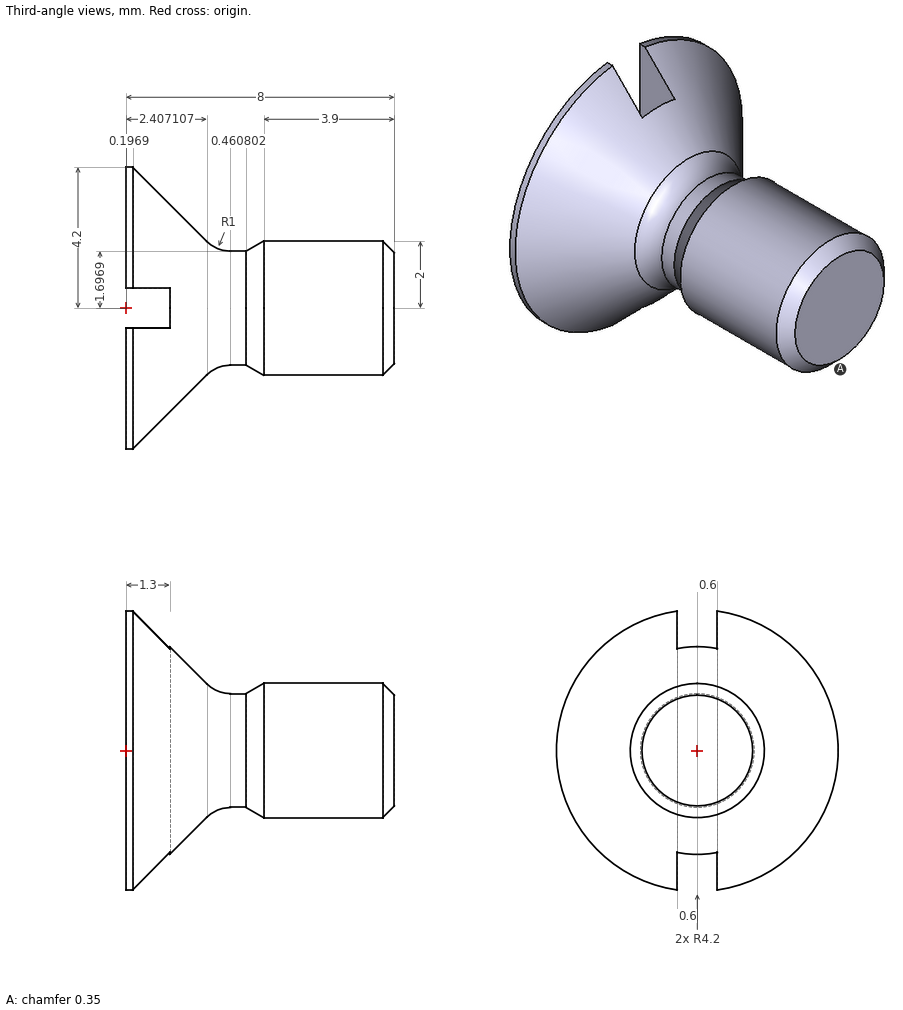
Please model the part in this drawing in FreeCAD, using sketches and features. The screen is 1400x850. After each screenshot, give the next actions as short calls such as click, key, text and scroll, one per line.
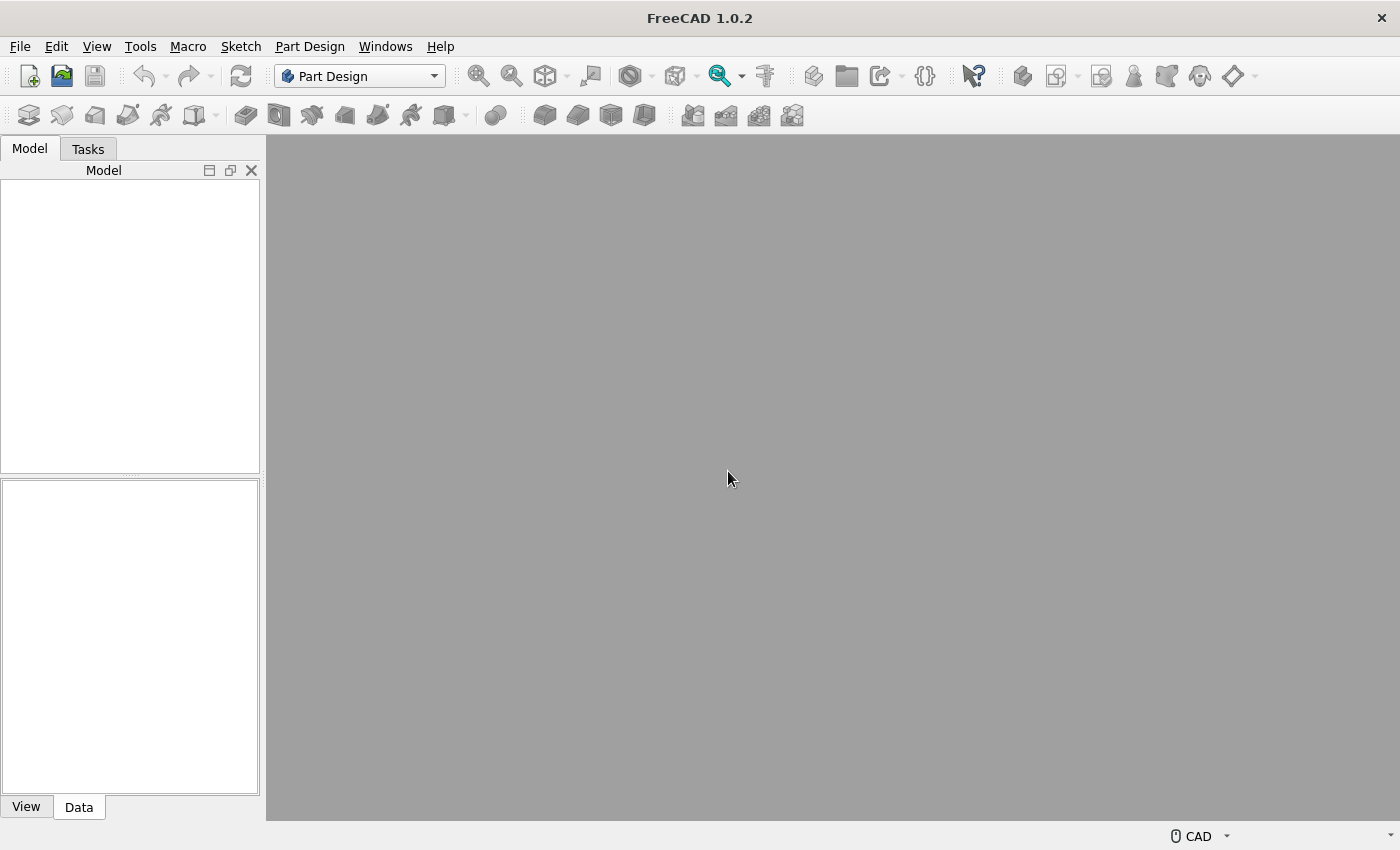
key(ctrl+n)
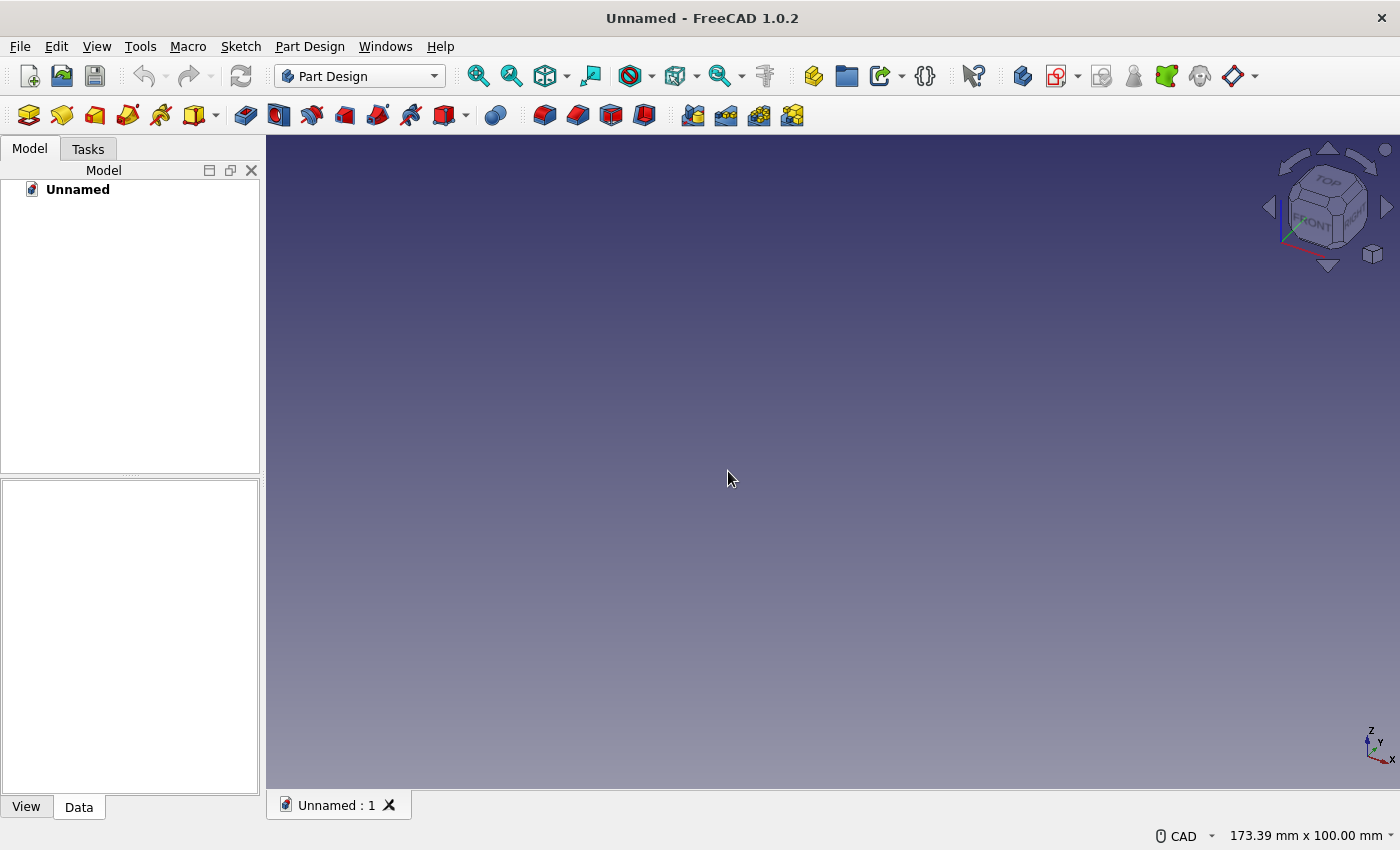
click(1056, 76)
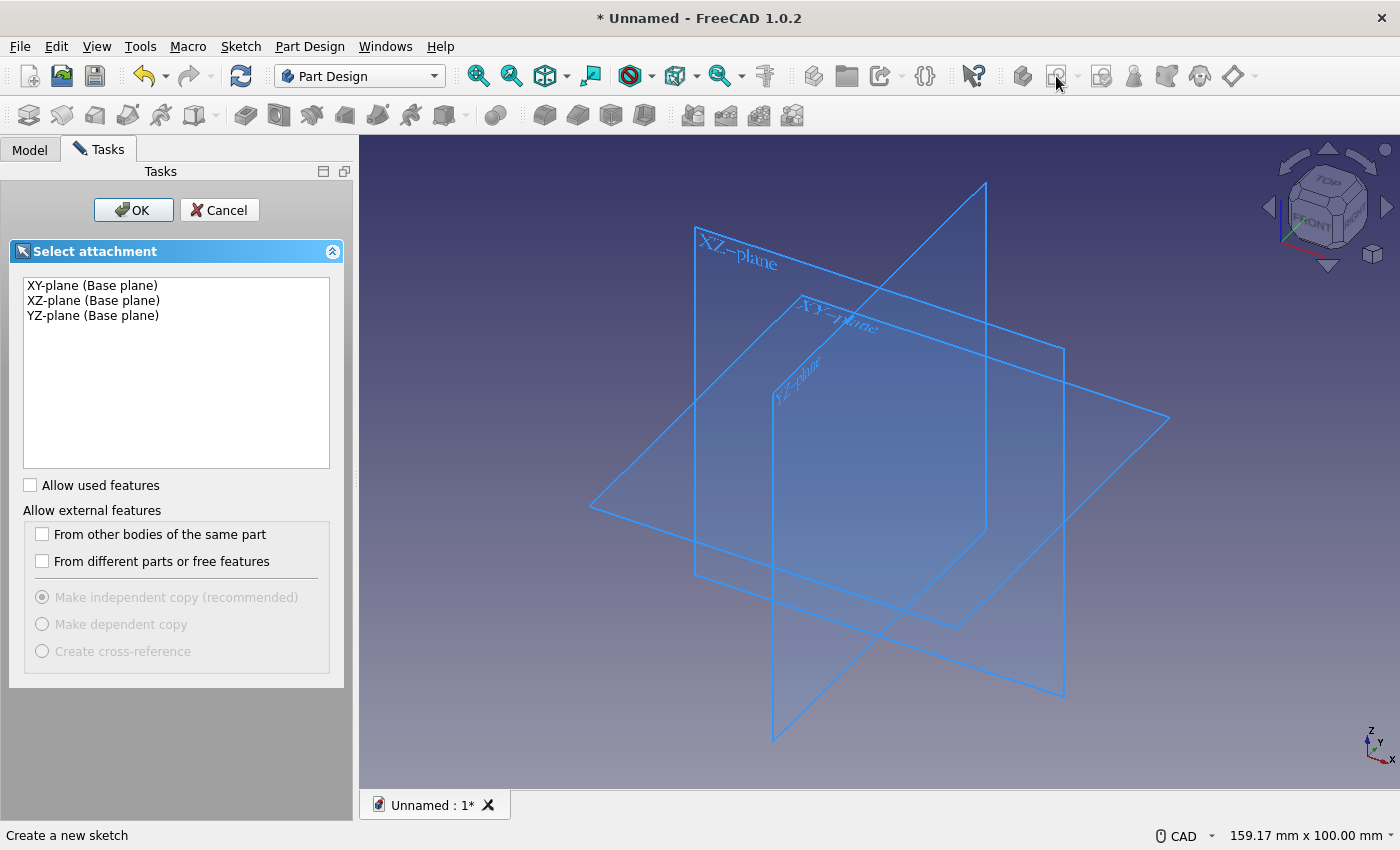
click(84, 286)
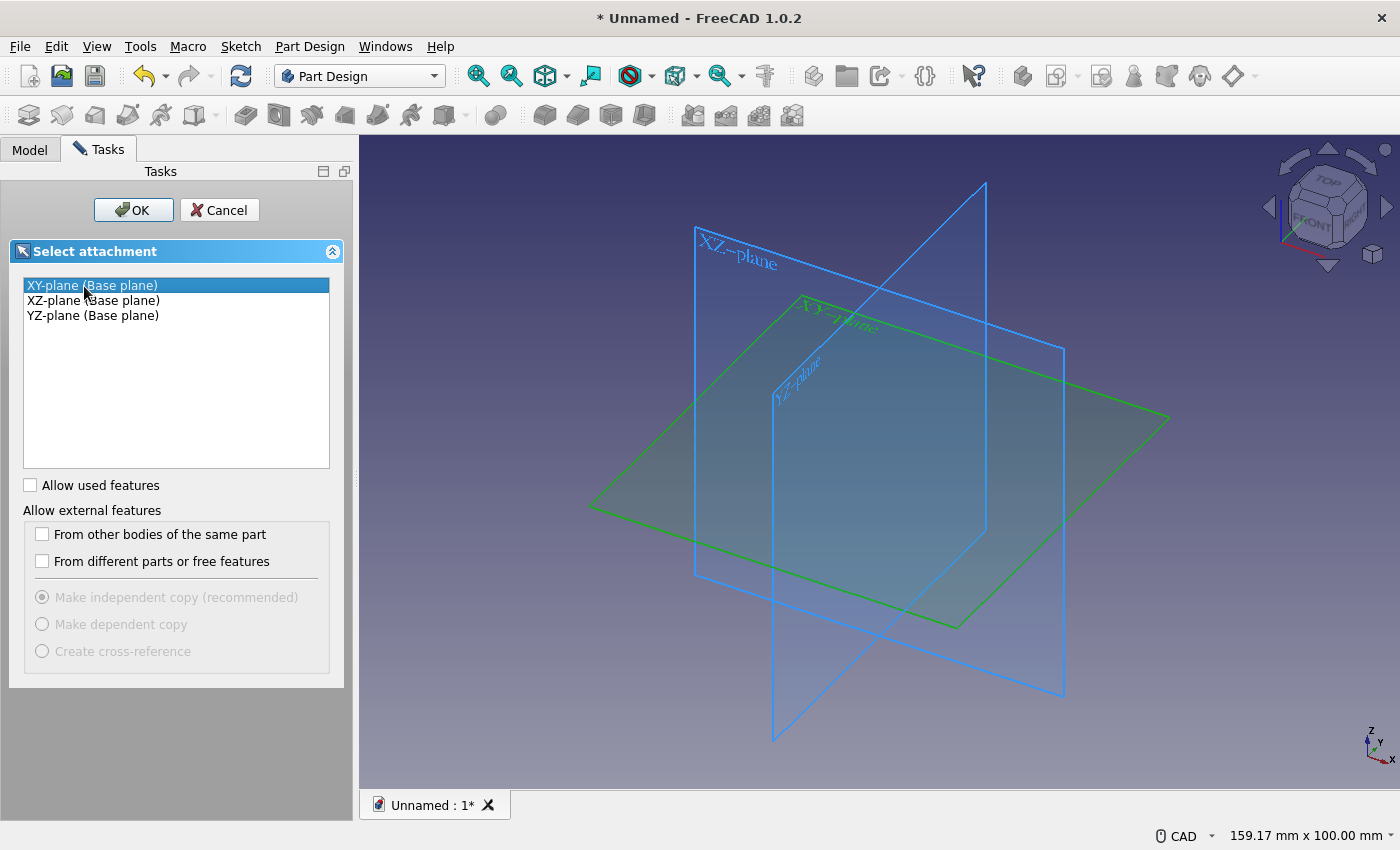
click(134, 210)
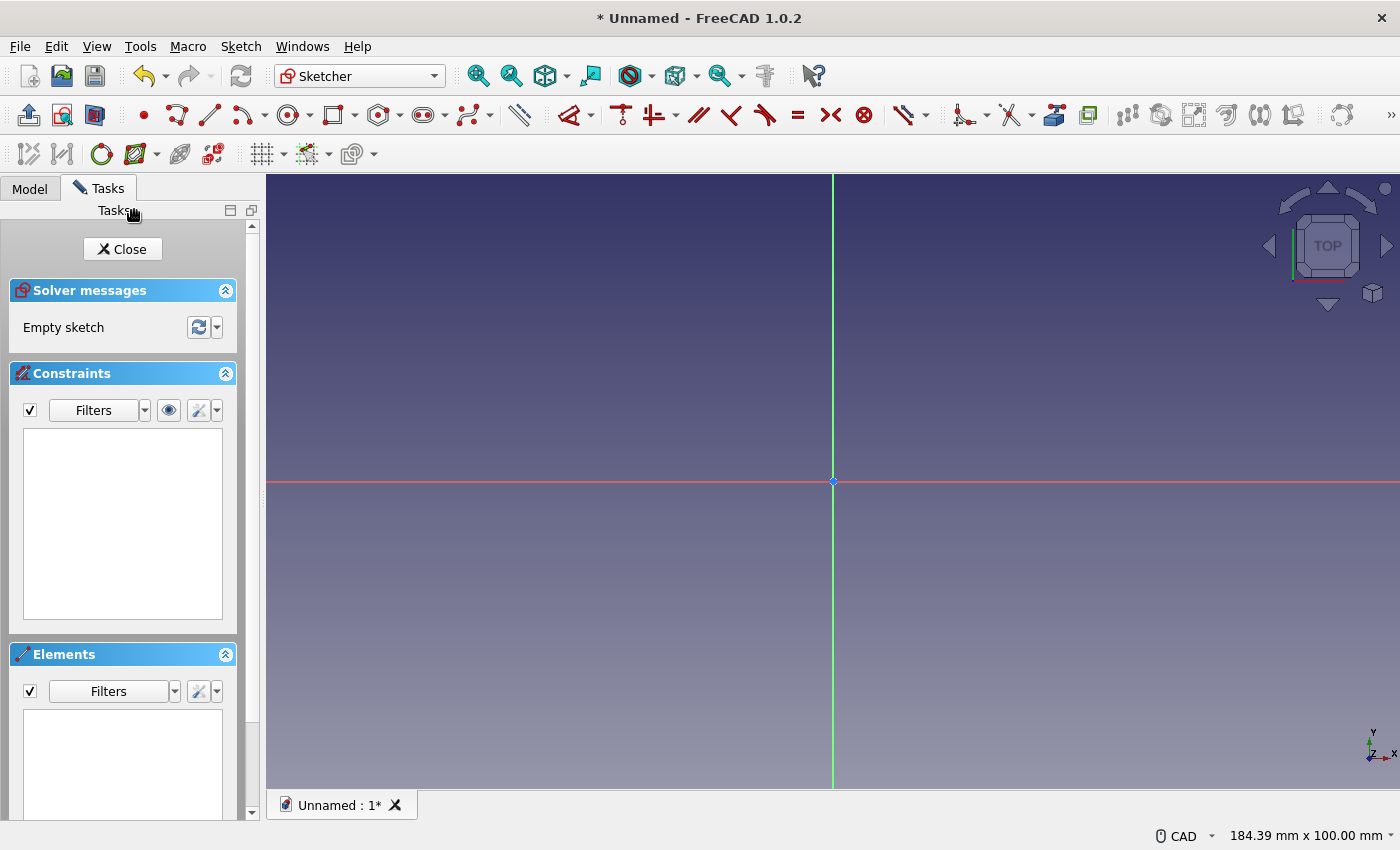
scroll(865, 468, up, 13)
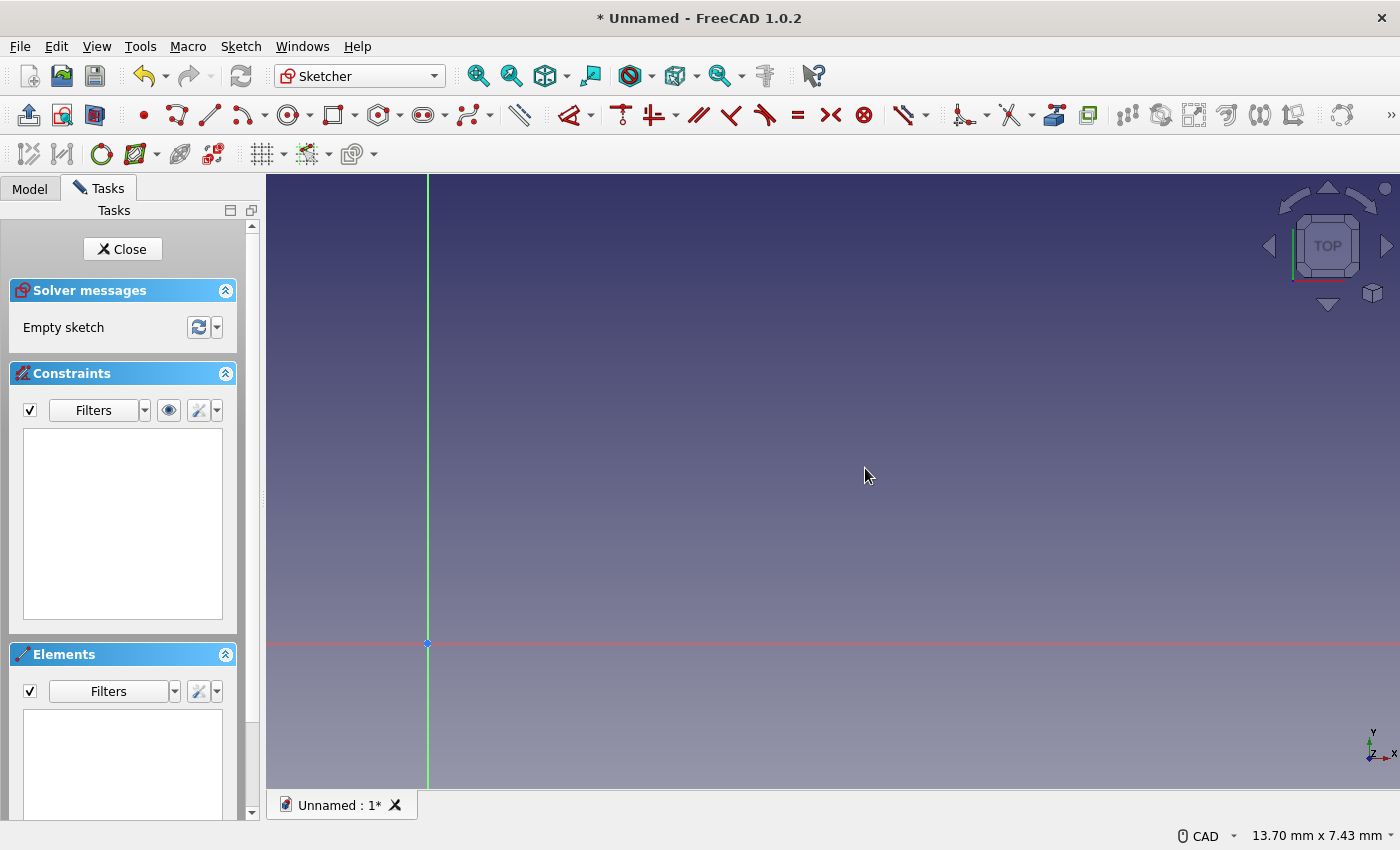
click(177, 116)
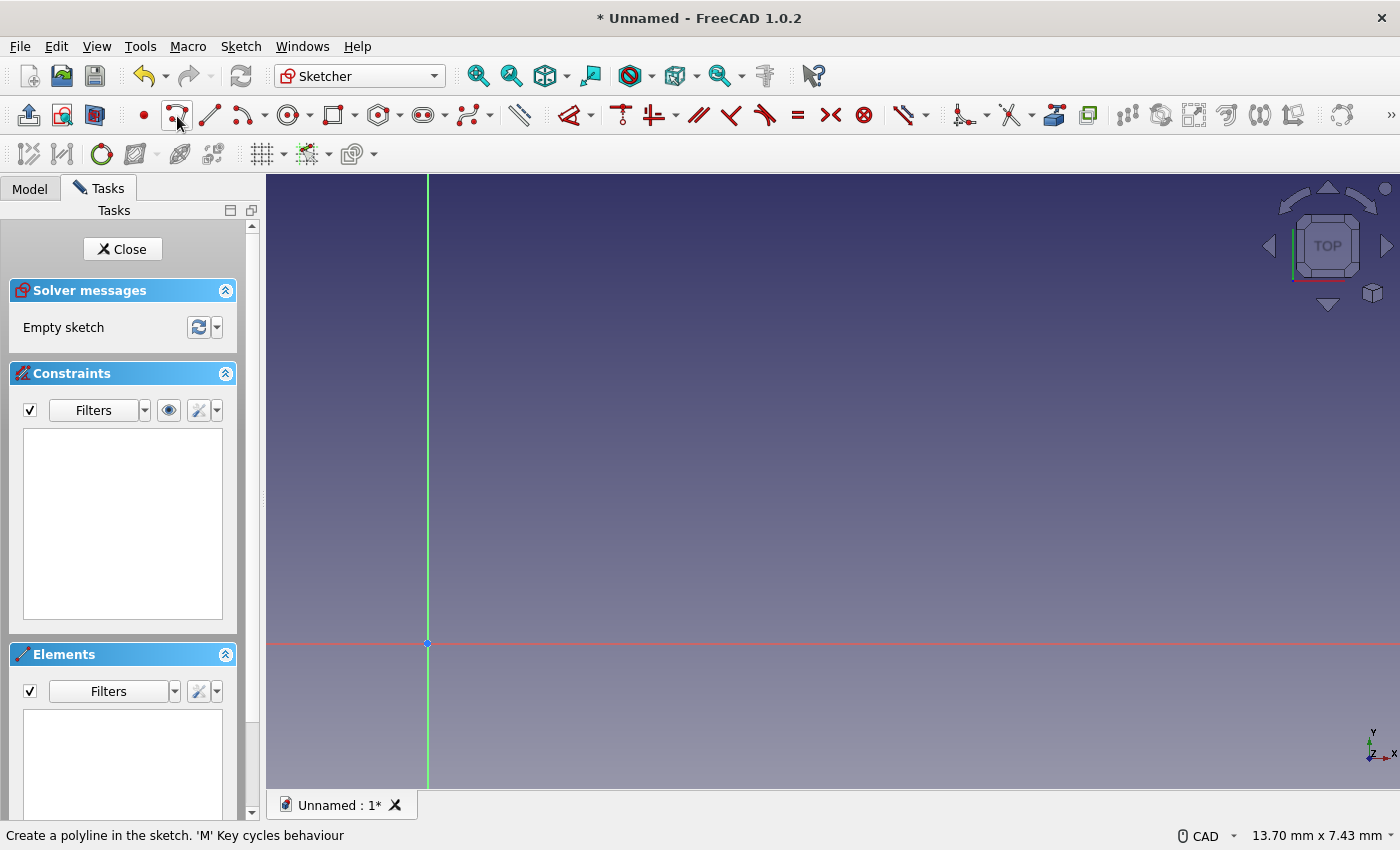
click(627, 479)
click(444, 296)
click(428, 296)
click(428, 644)
click(1090, 635)
click(1090, 478)
click(767, 478)
click(724, 503)
click(685, 503)
right_click(685, 503)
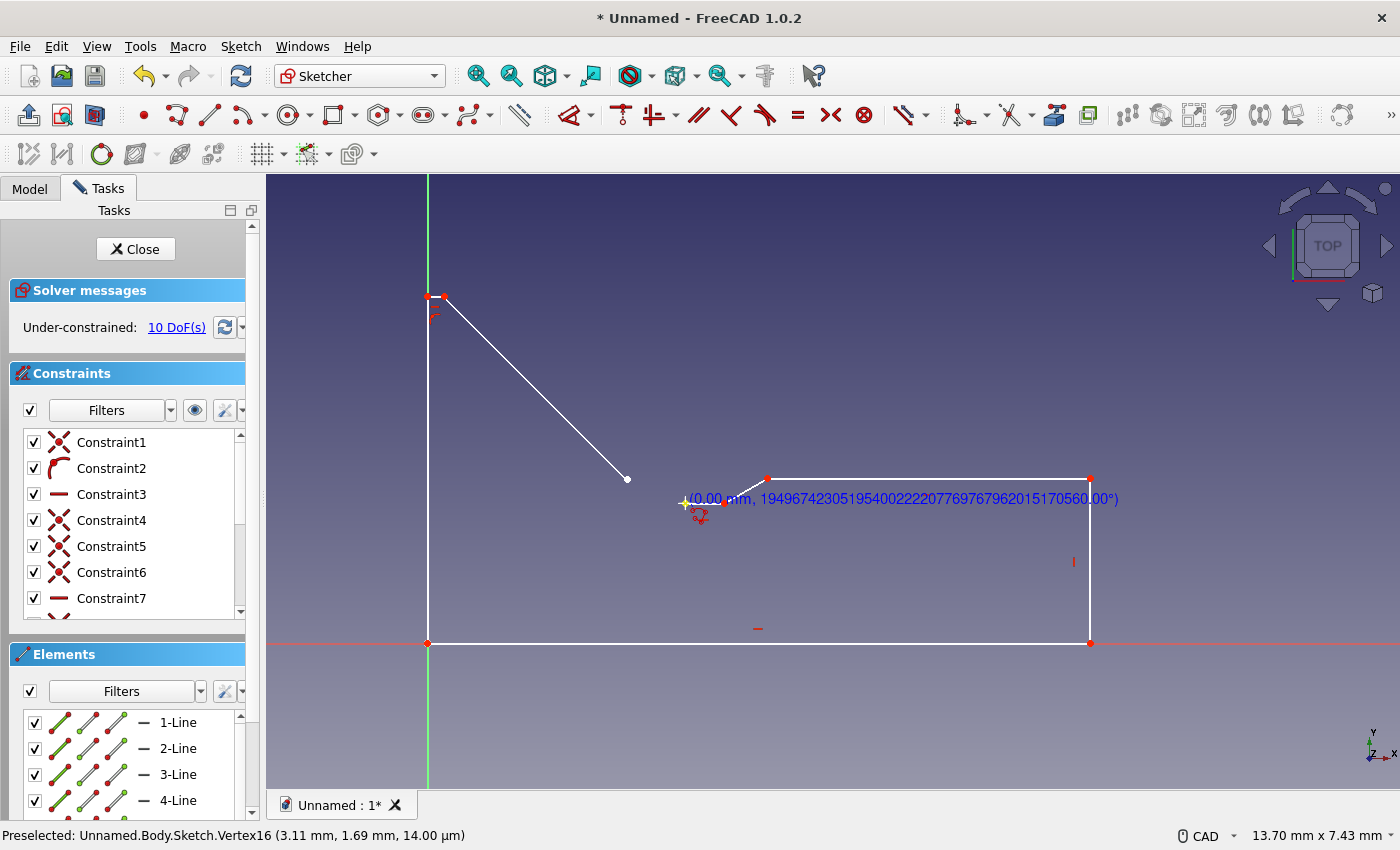
key(g)
key(3)
key(a)